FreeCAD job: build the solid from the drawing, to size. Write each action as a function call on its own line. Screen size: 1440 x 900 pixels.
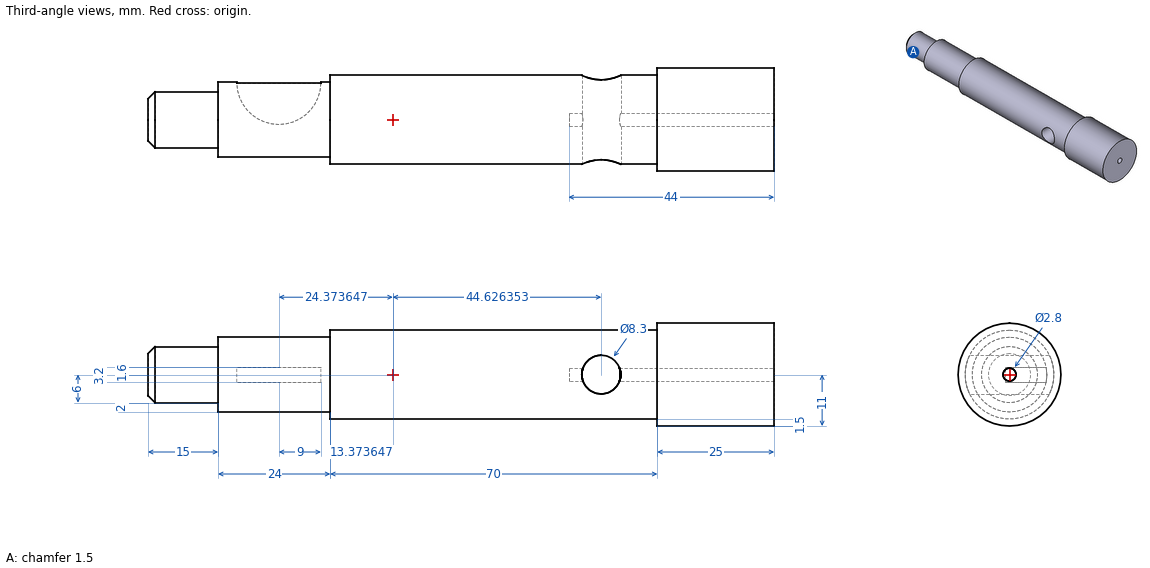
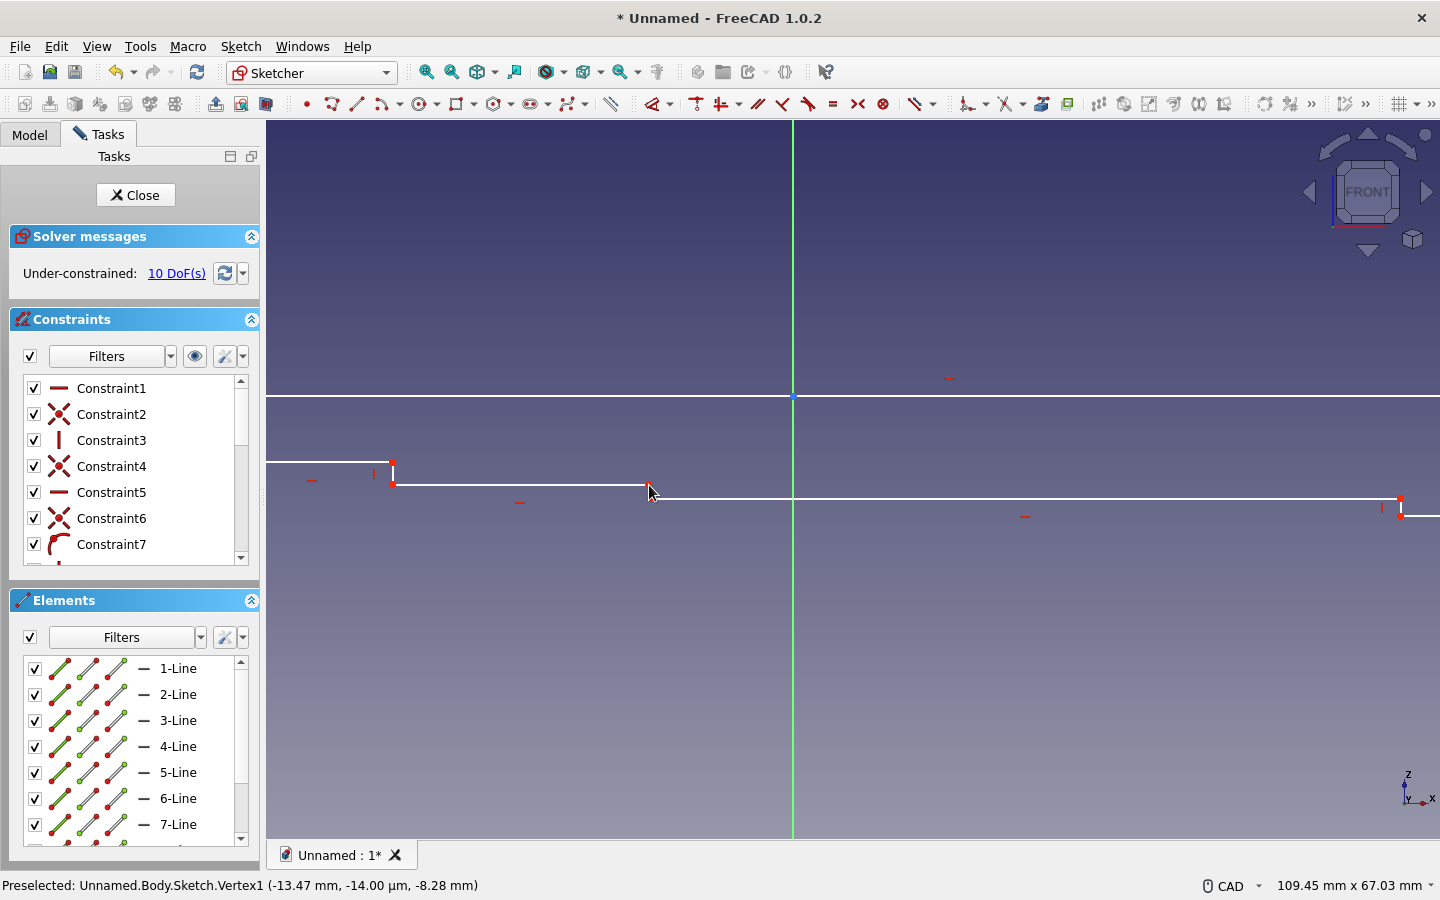
scroll(649, 492, up, 4)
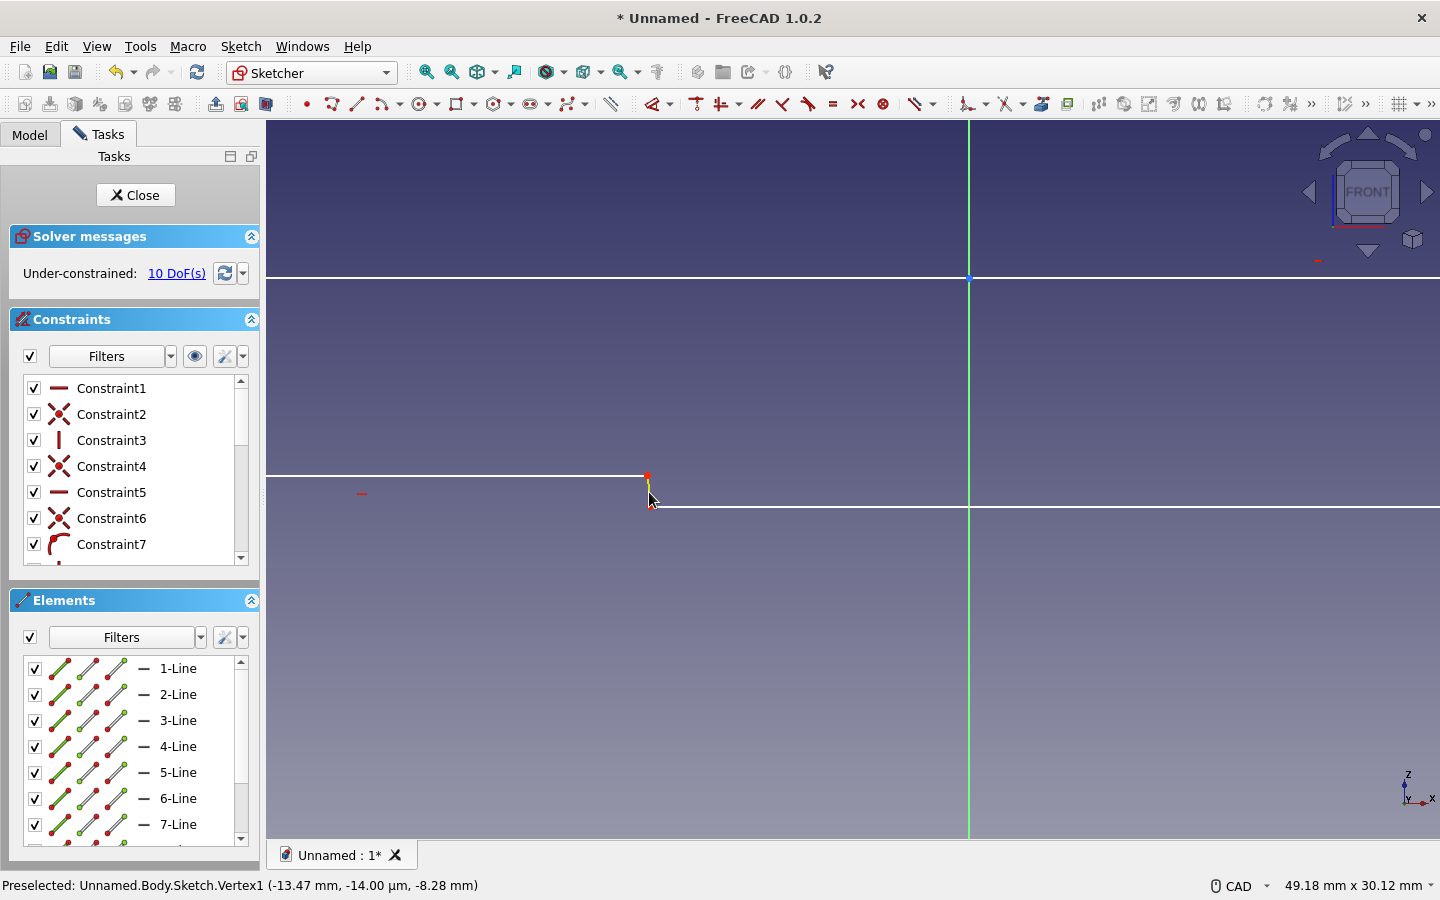
click(649, 491)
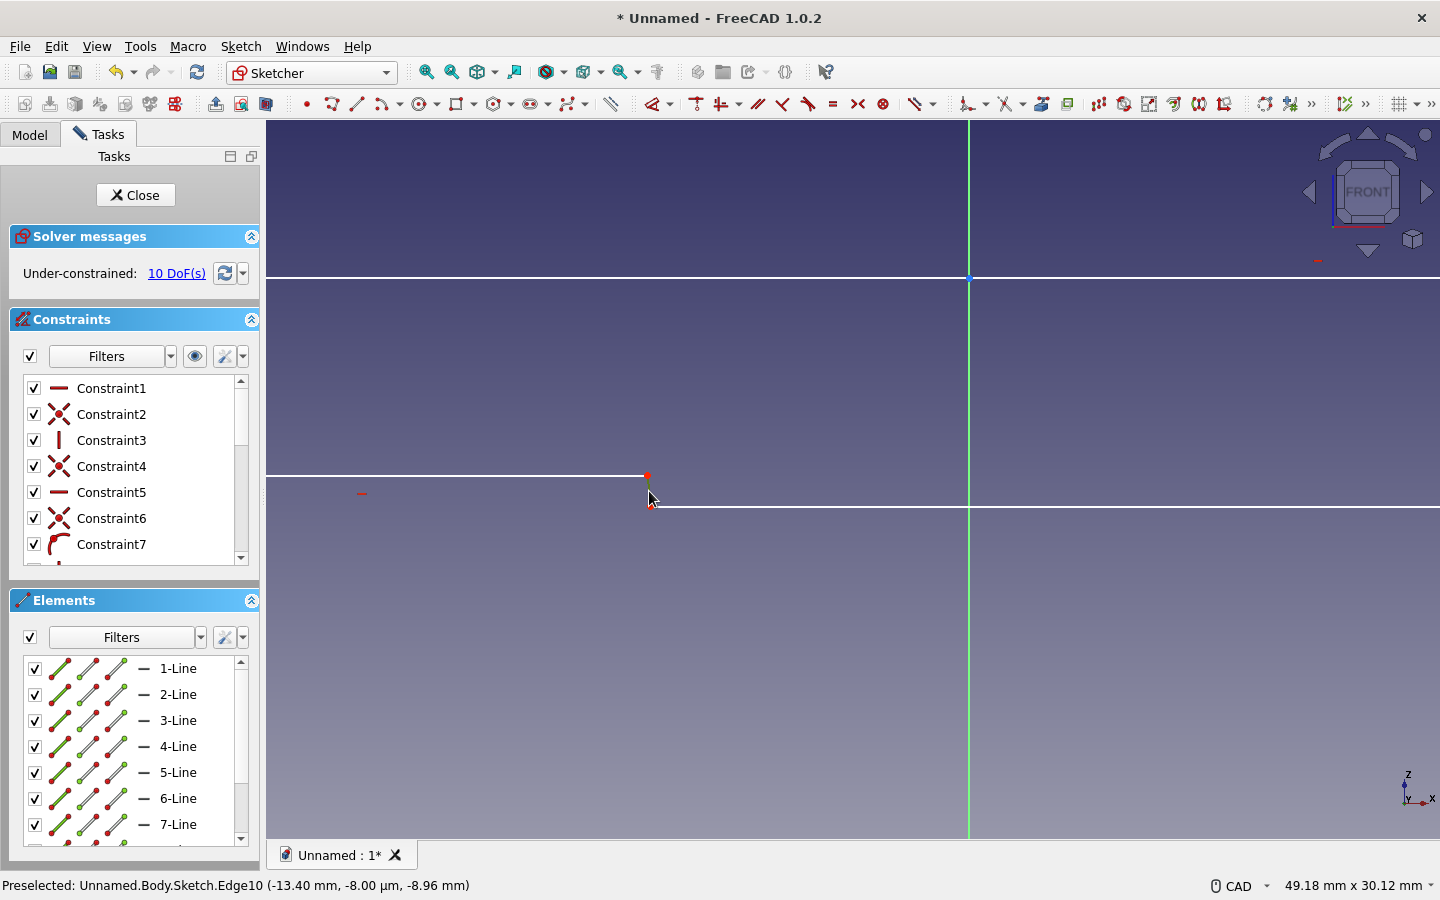
key(v)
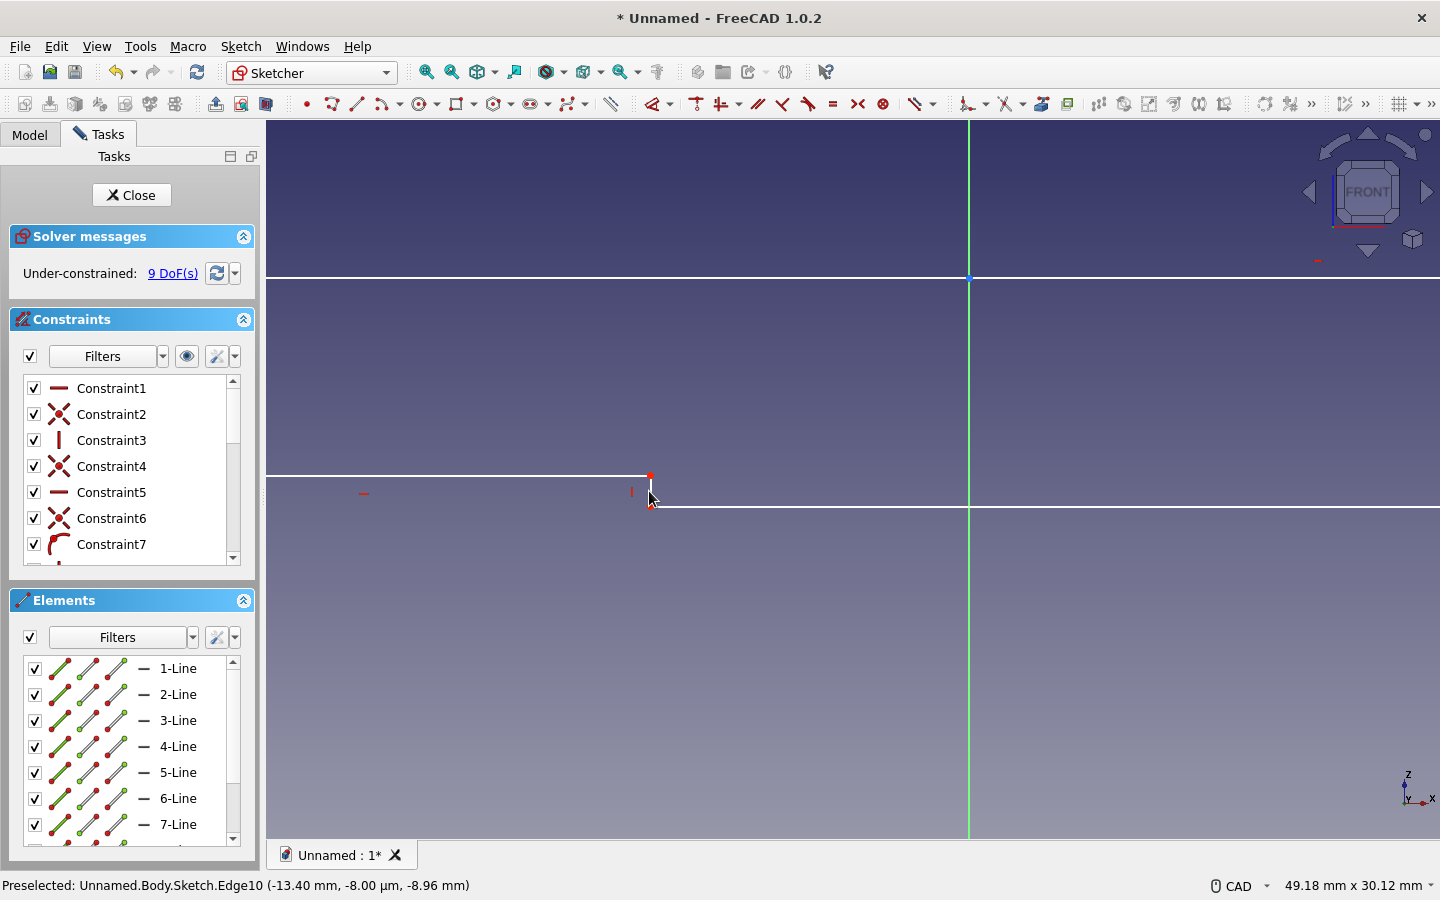
scroll(649, 497, down, 8)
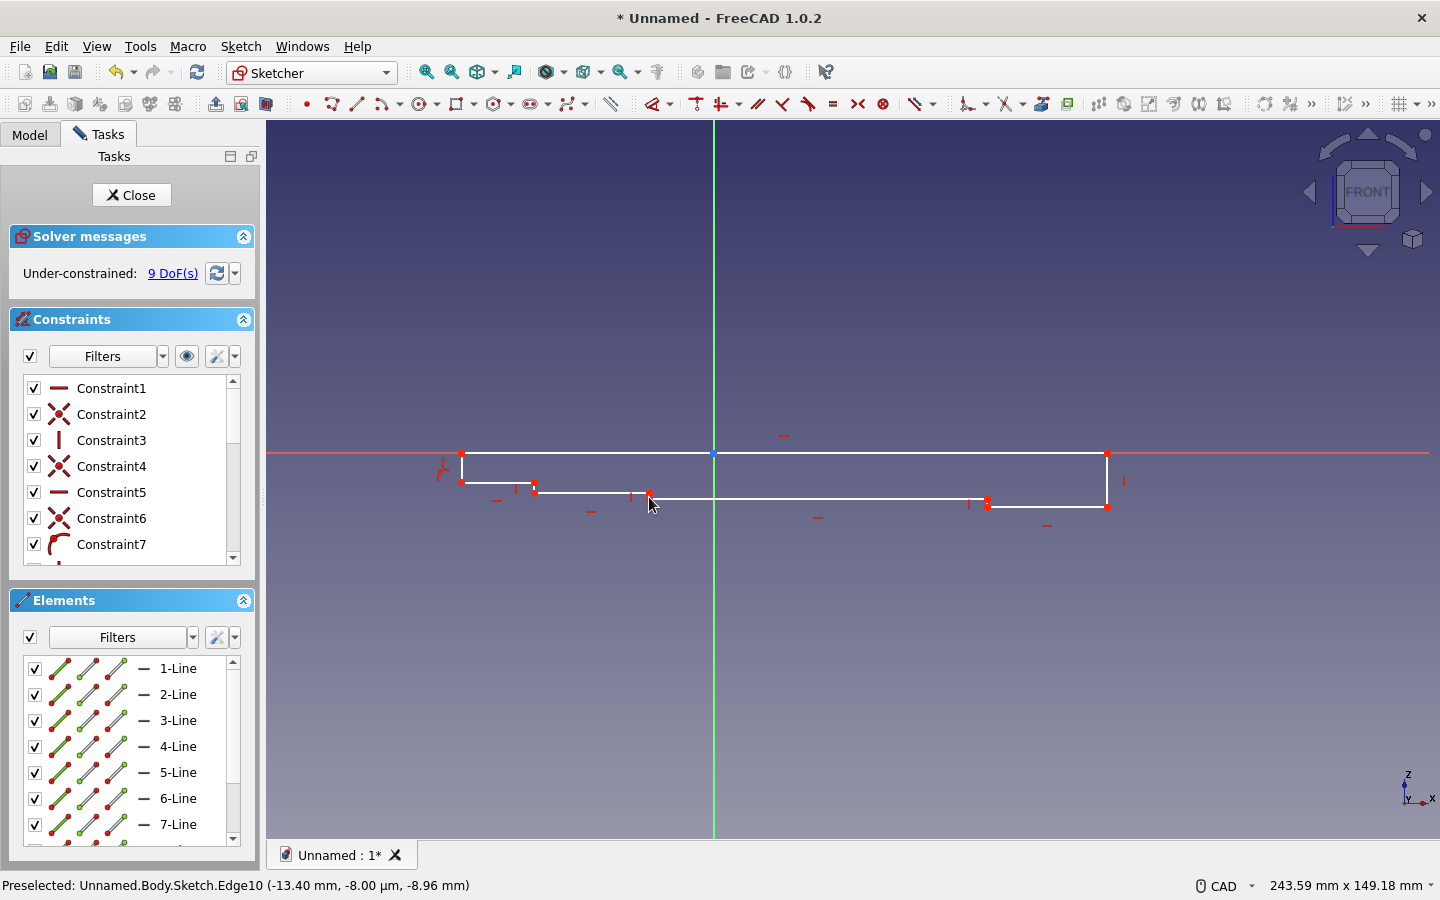
scroll(534, 490, up, 8)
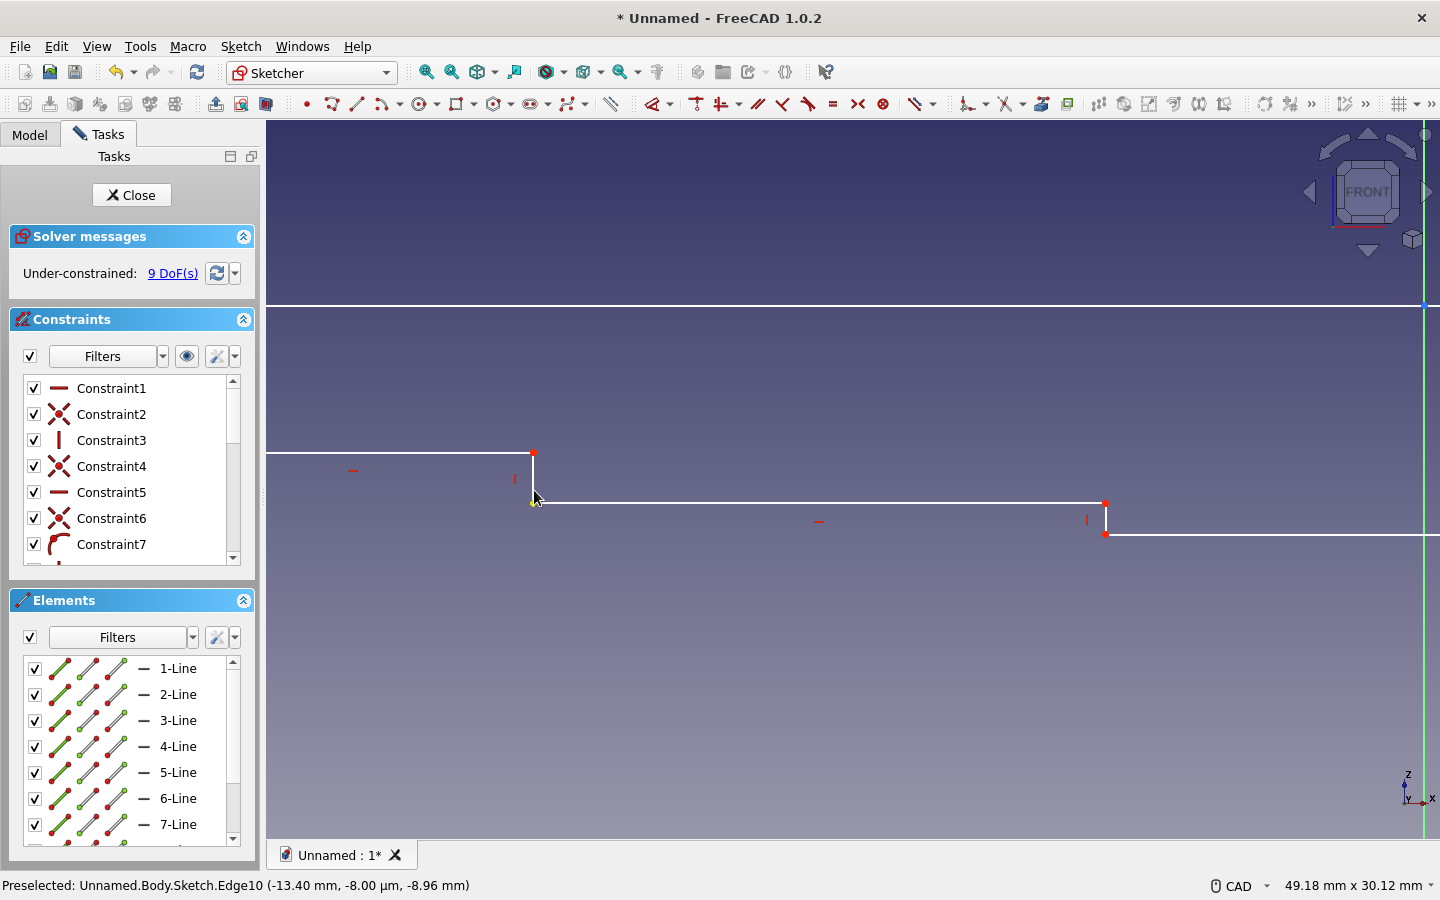
click(533, 488)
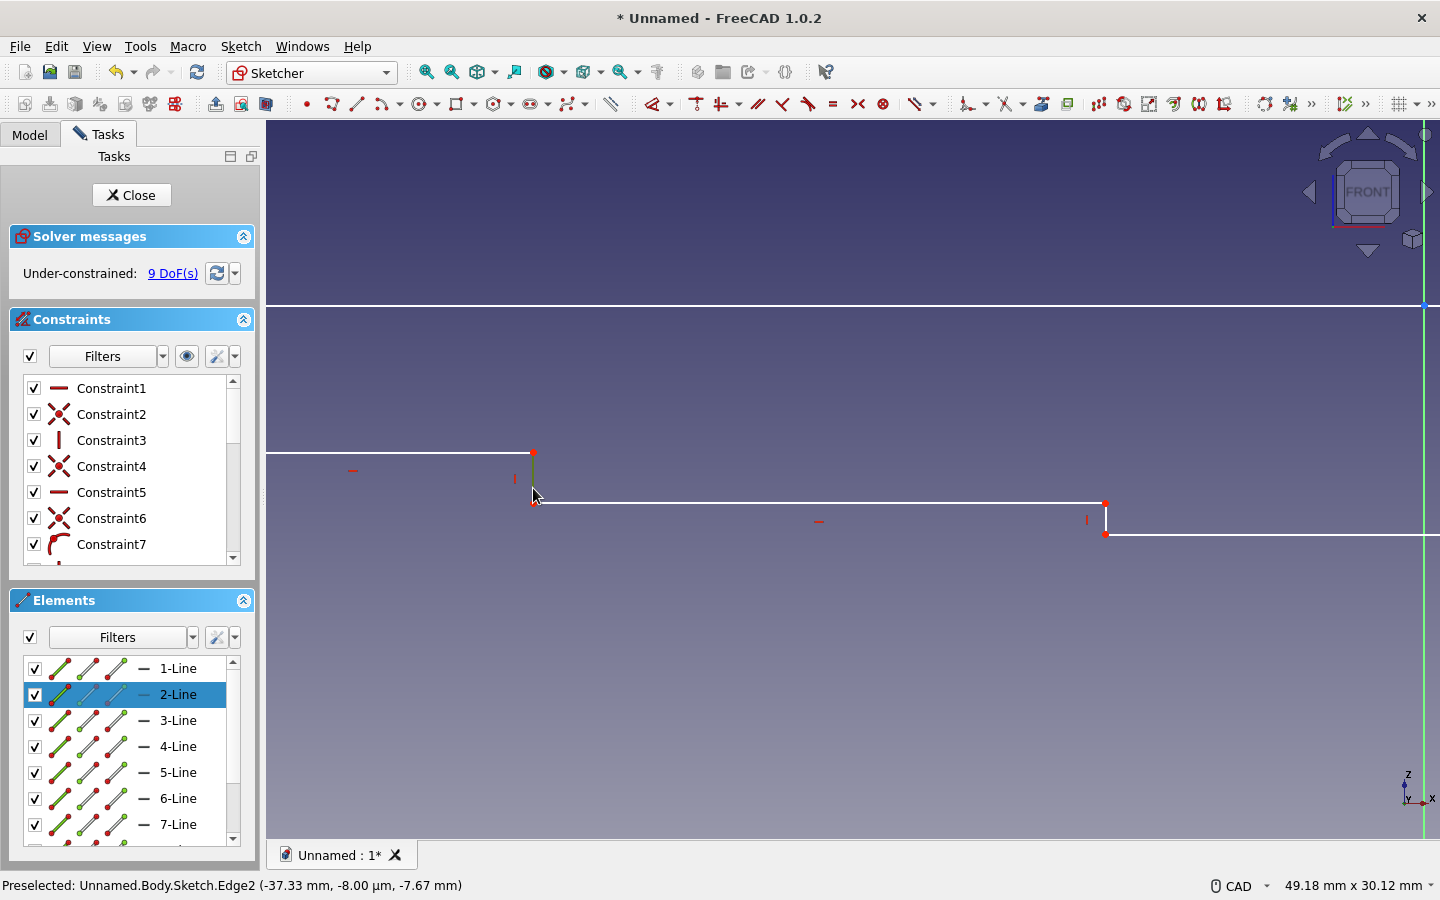
key(i)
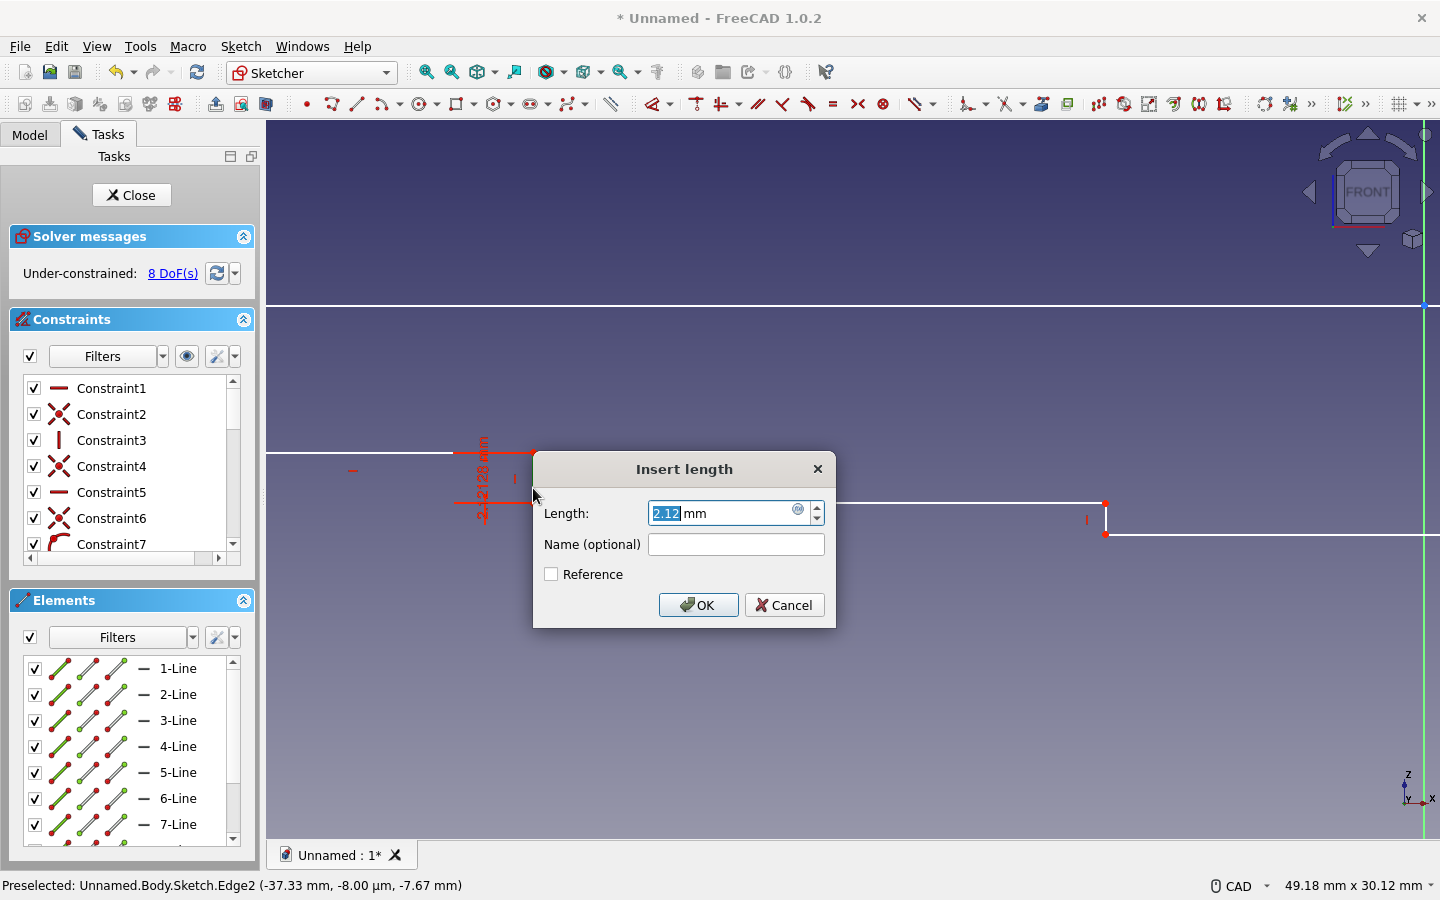
text(2)
key(Return)